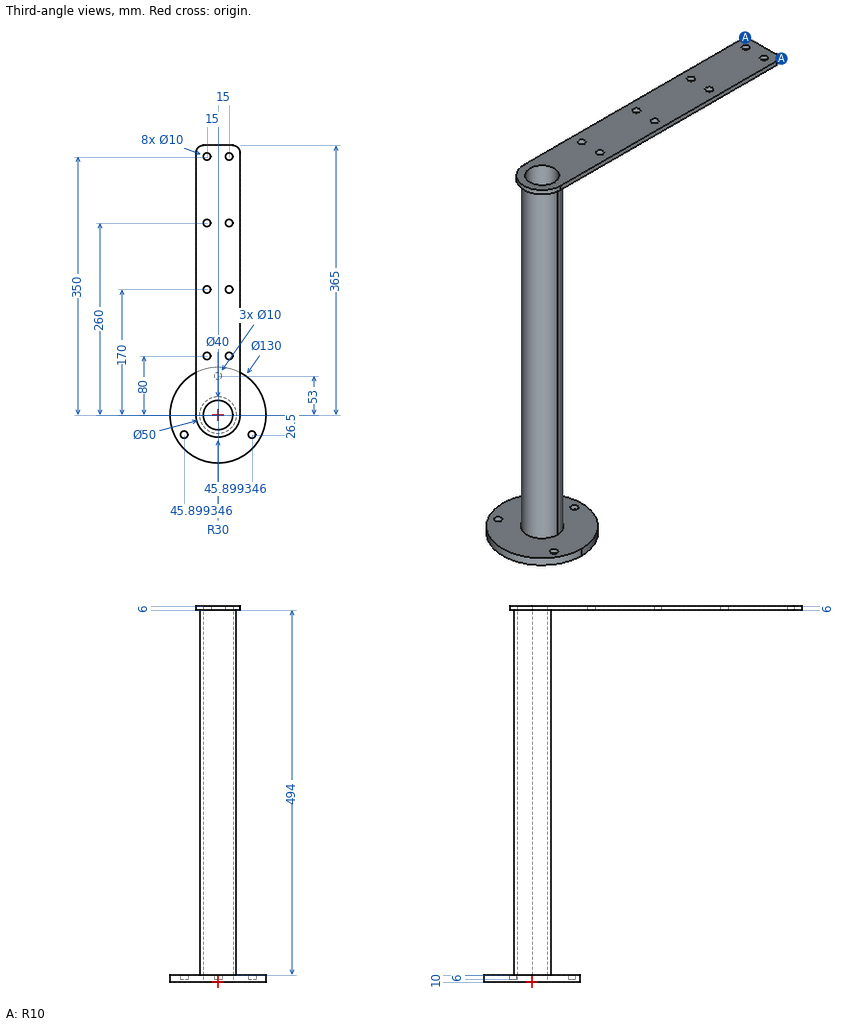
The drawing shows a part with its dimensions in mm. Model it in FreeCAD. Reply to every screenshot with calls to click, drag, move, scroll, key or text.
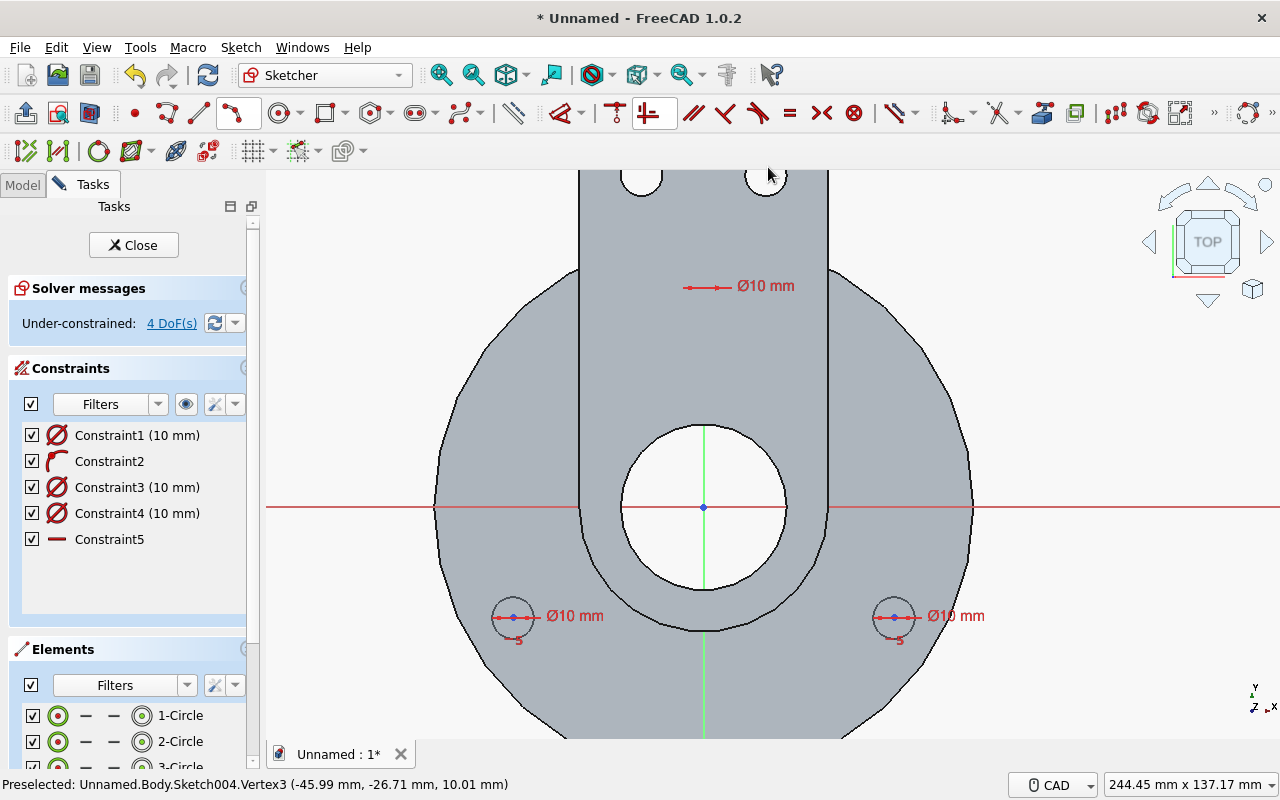
click(560, 114)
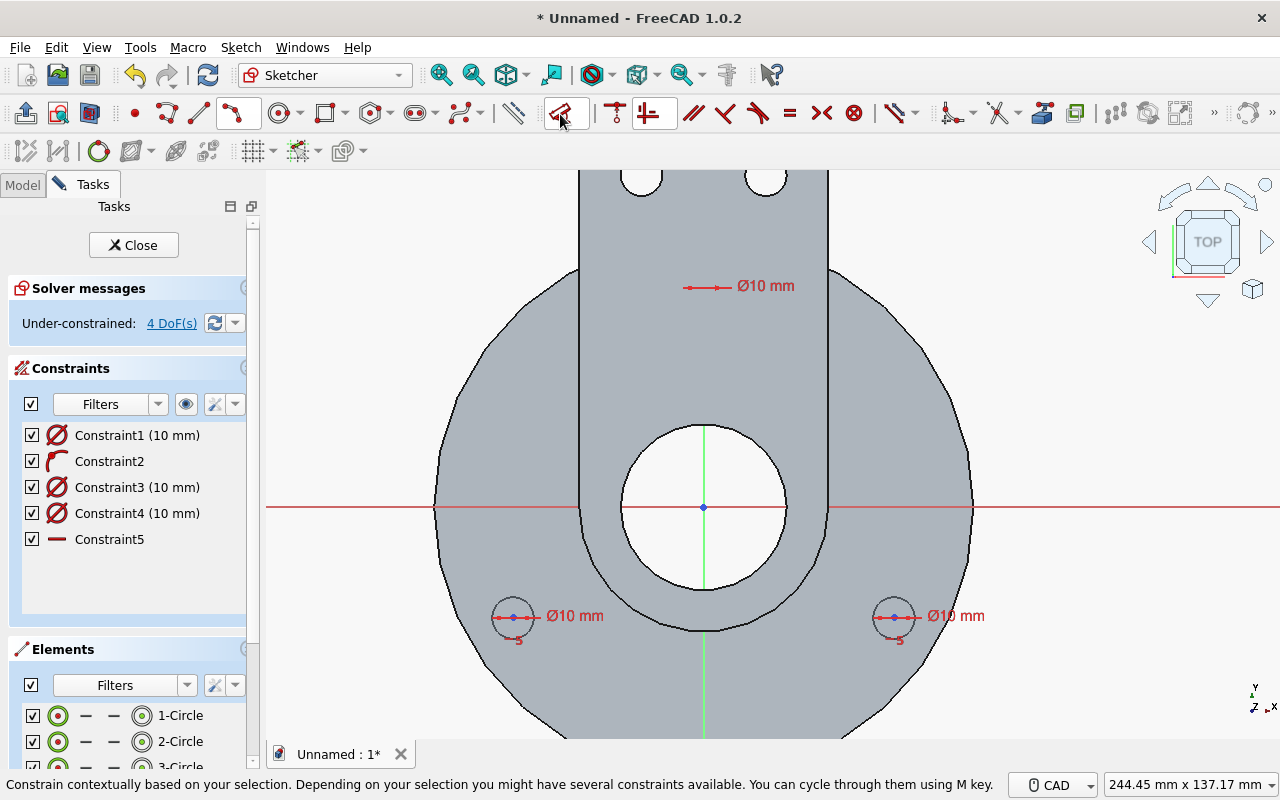
click(704, 288)
click(738, 398)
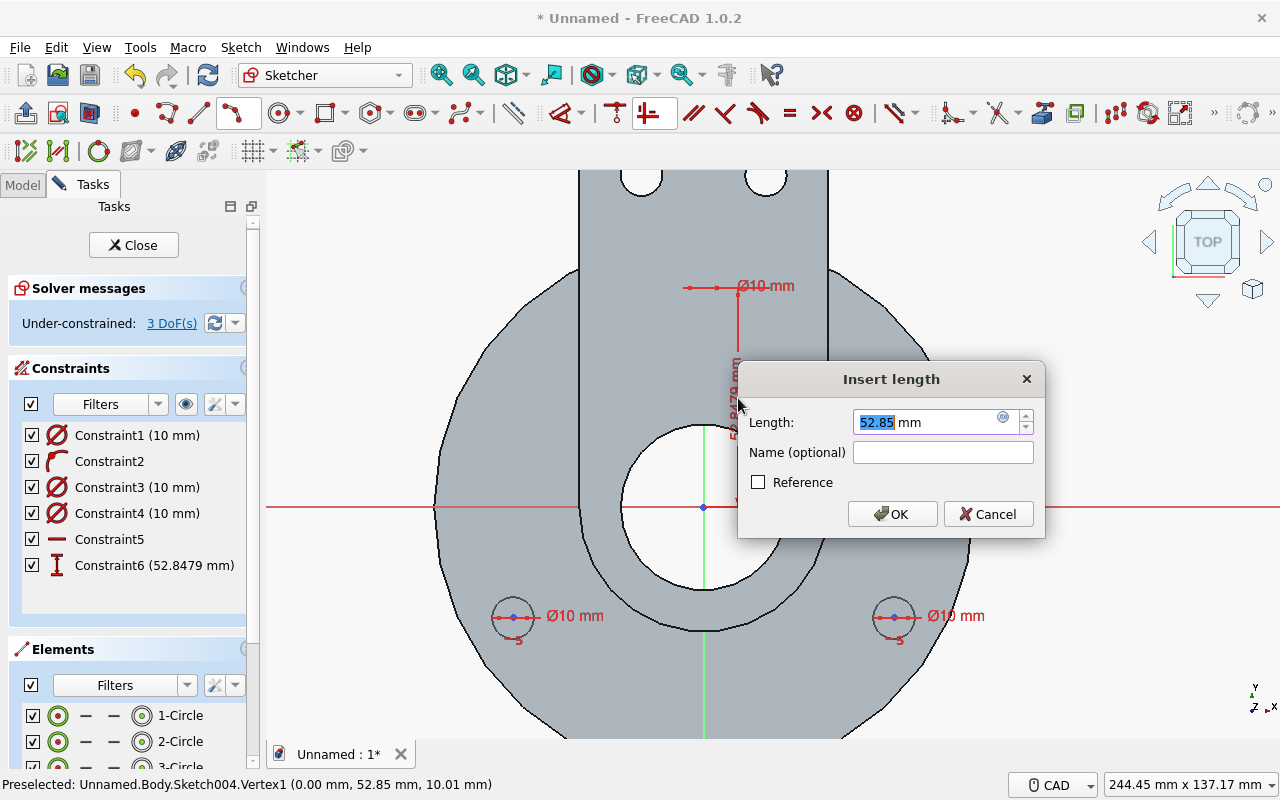
text(53)
key(Return)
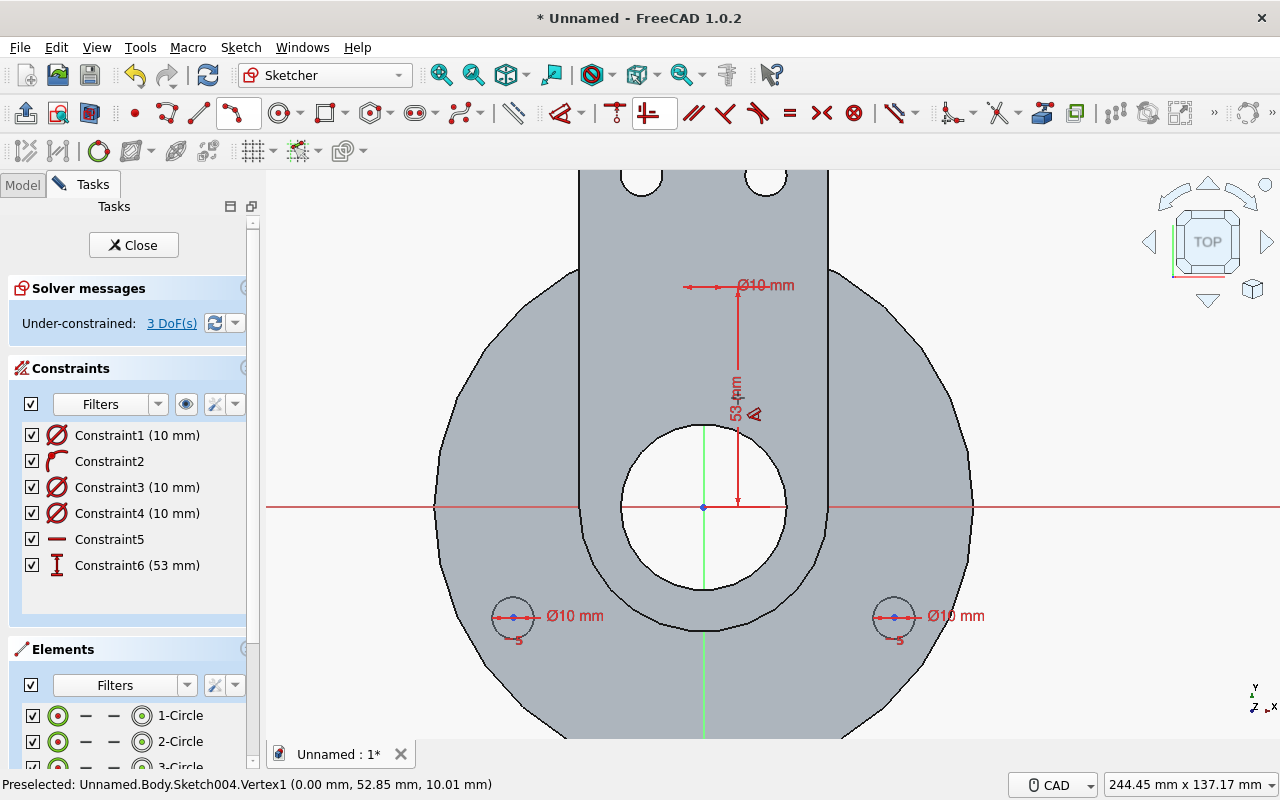
click(894, 618)
click(928, 563)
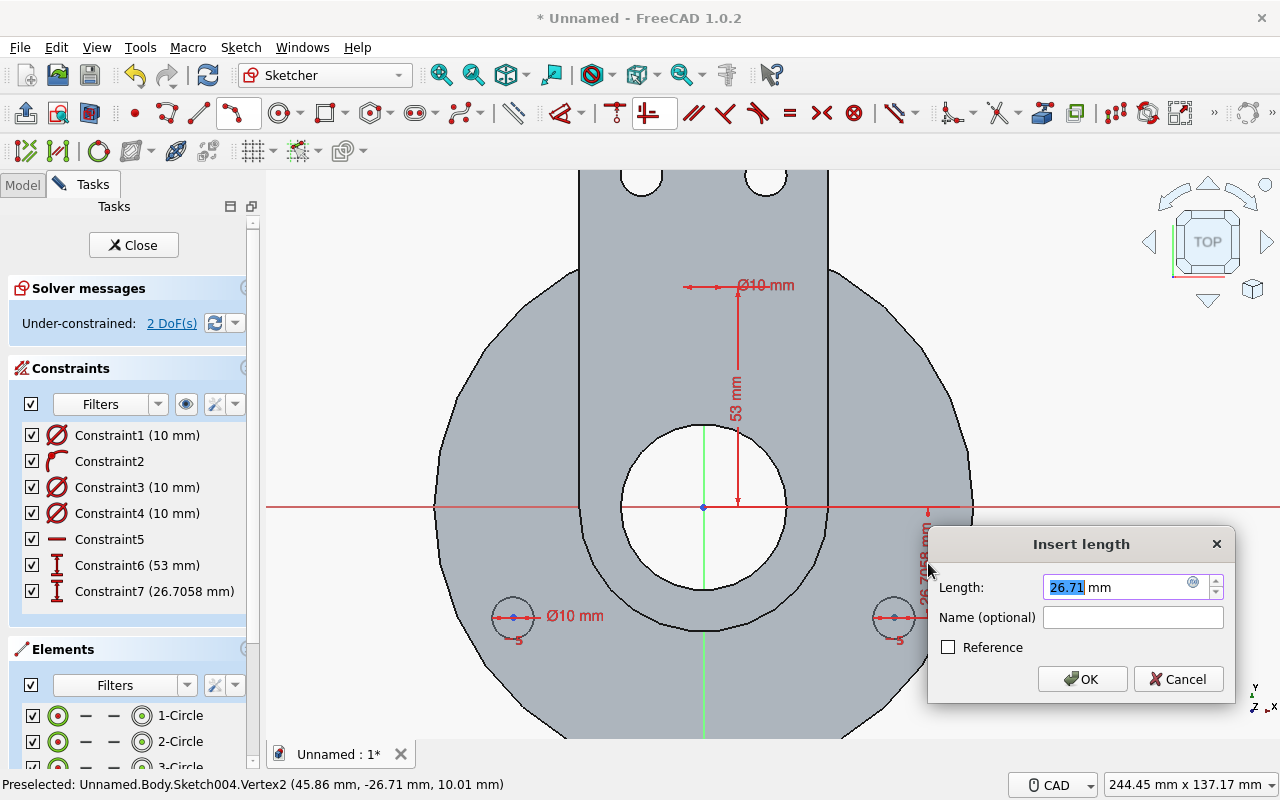
text(26.5)
key(Return)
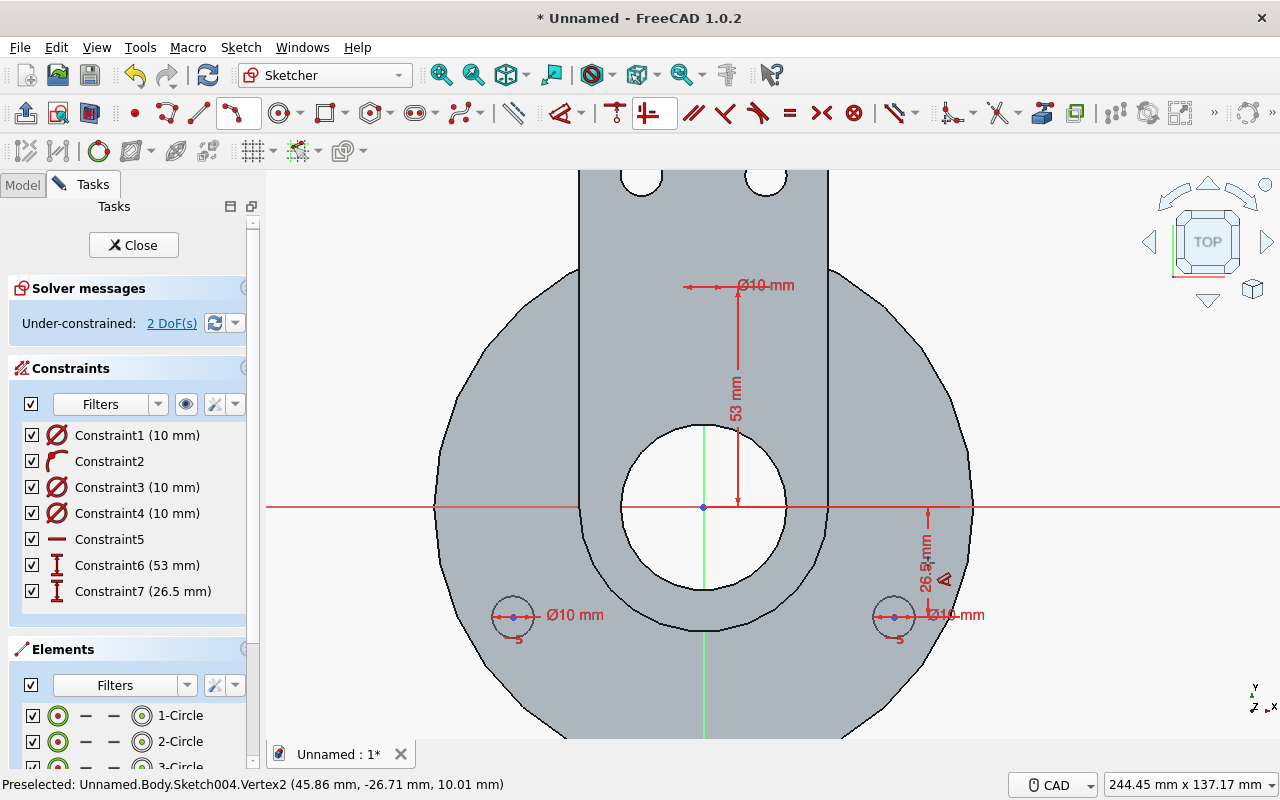
click(894, 617)
click(799, 651)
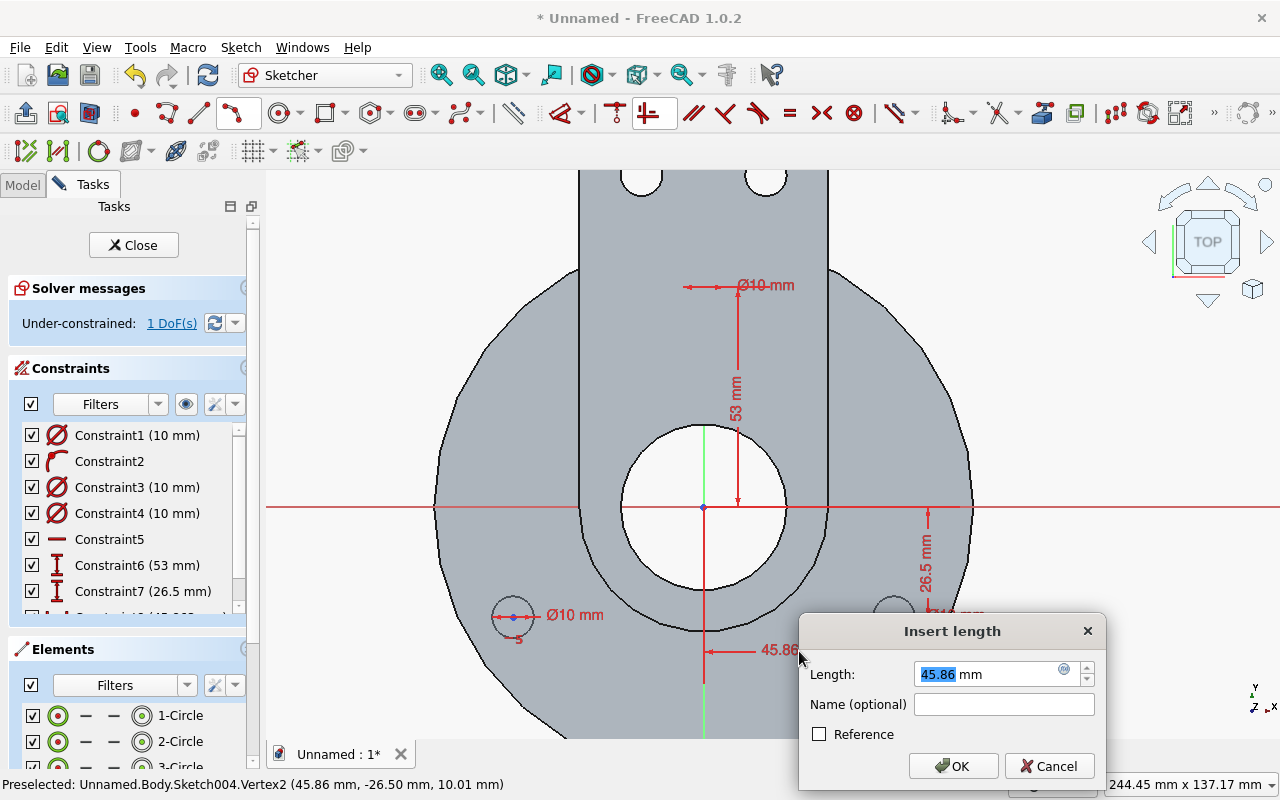
text(45.899346)
key(Return)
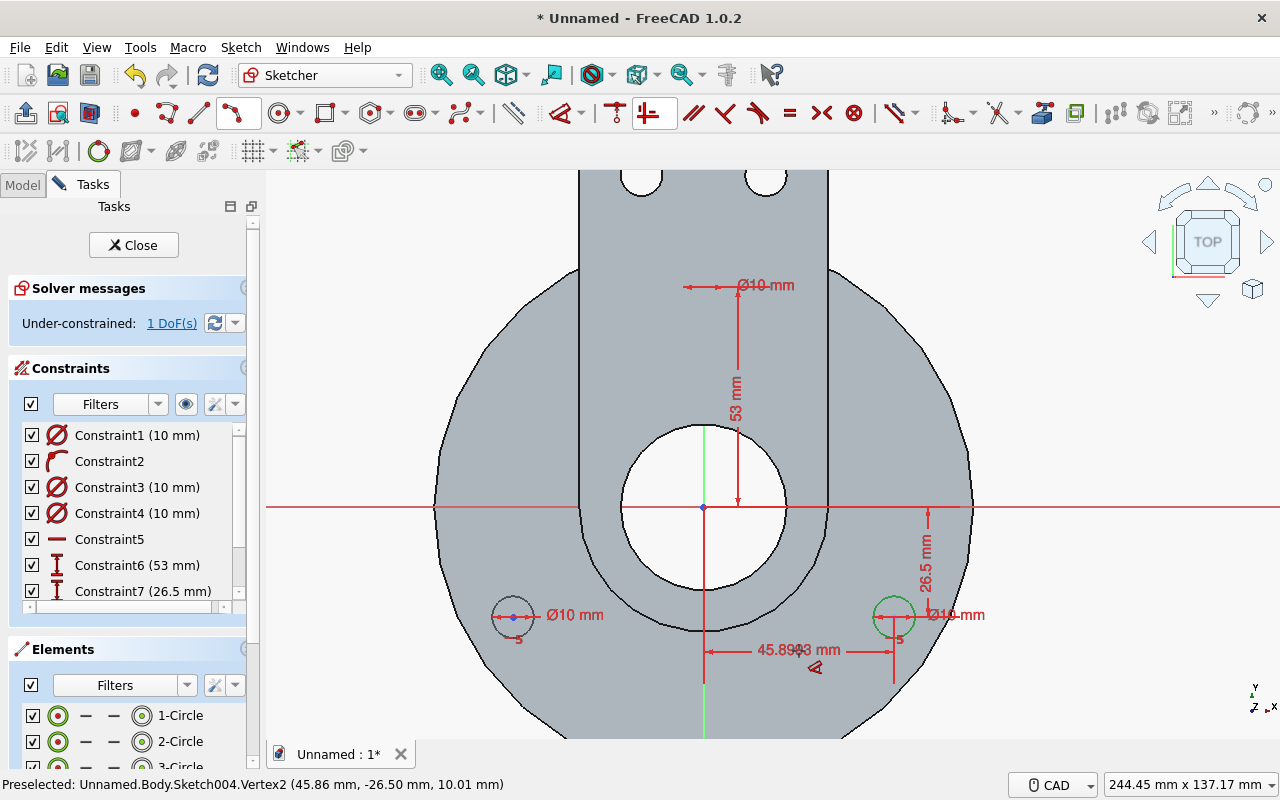
click(513, 617)
click(608, 651)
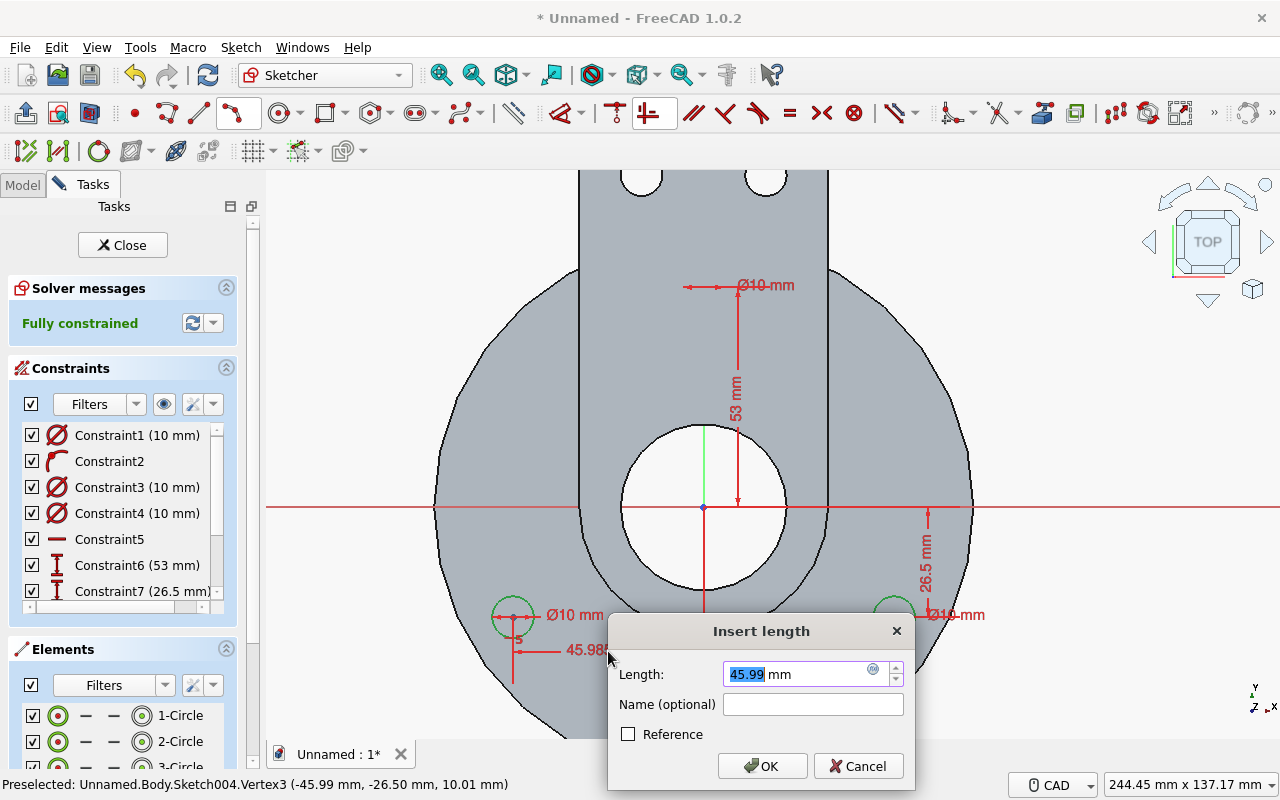
text(45.899346)
key(Return)
key(Escape)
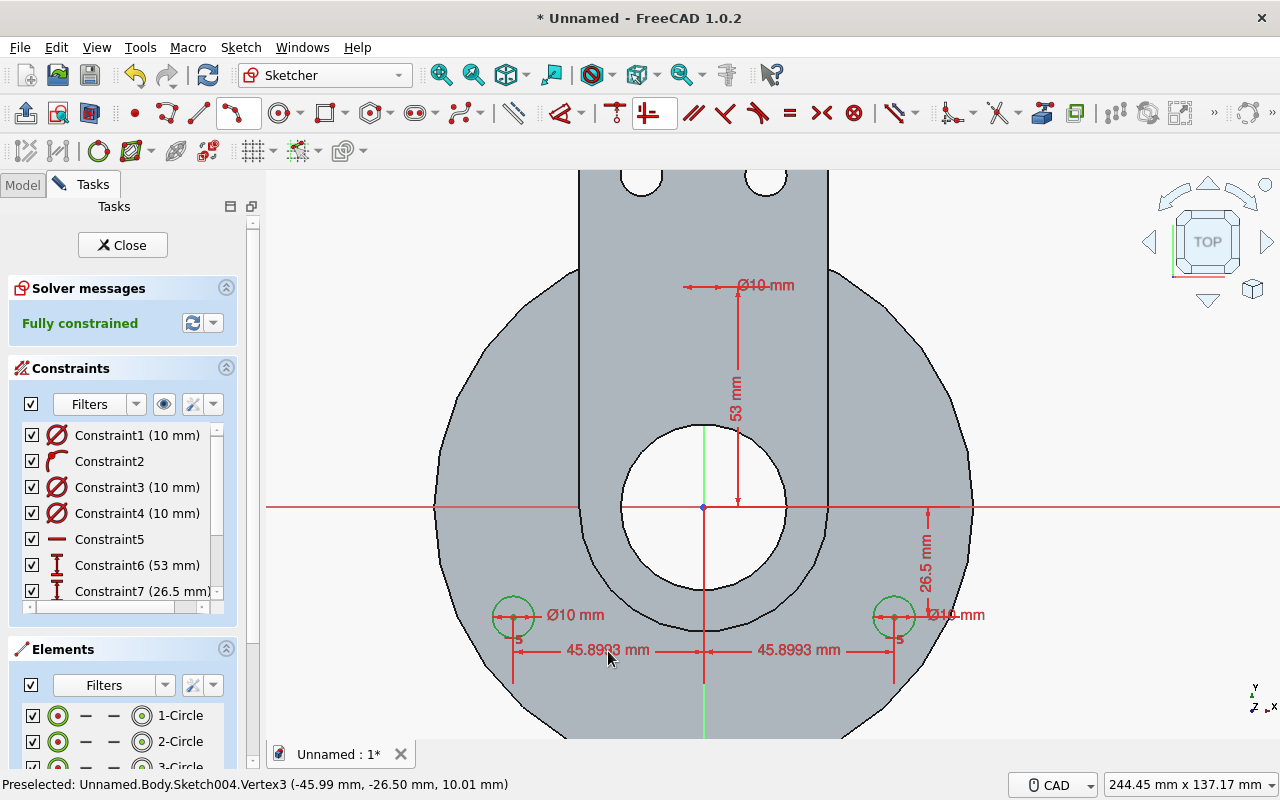
click(123, 245)